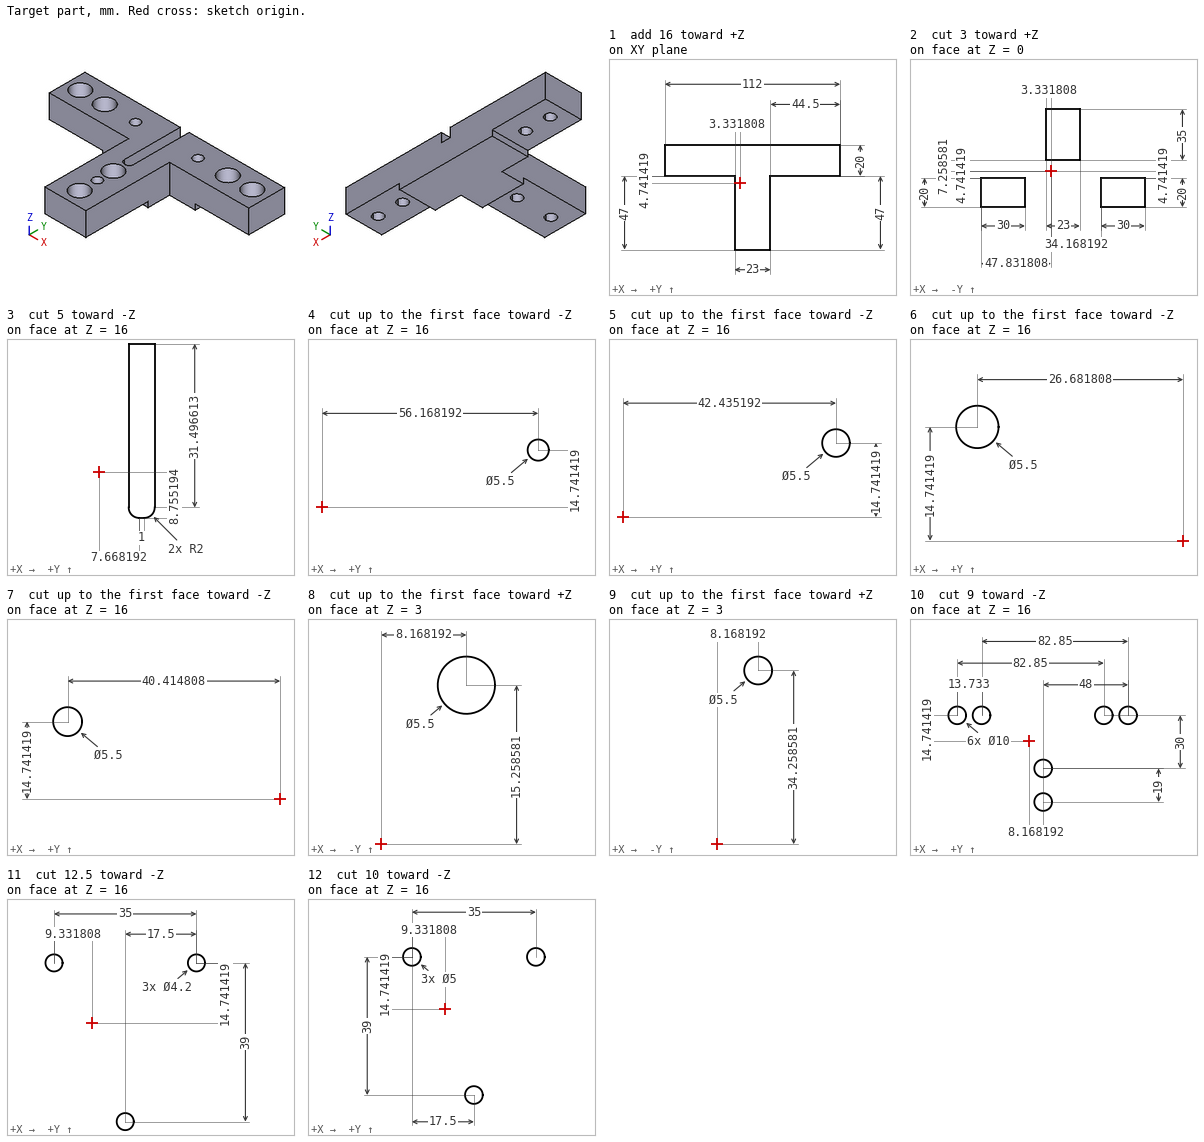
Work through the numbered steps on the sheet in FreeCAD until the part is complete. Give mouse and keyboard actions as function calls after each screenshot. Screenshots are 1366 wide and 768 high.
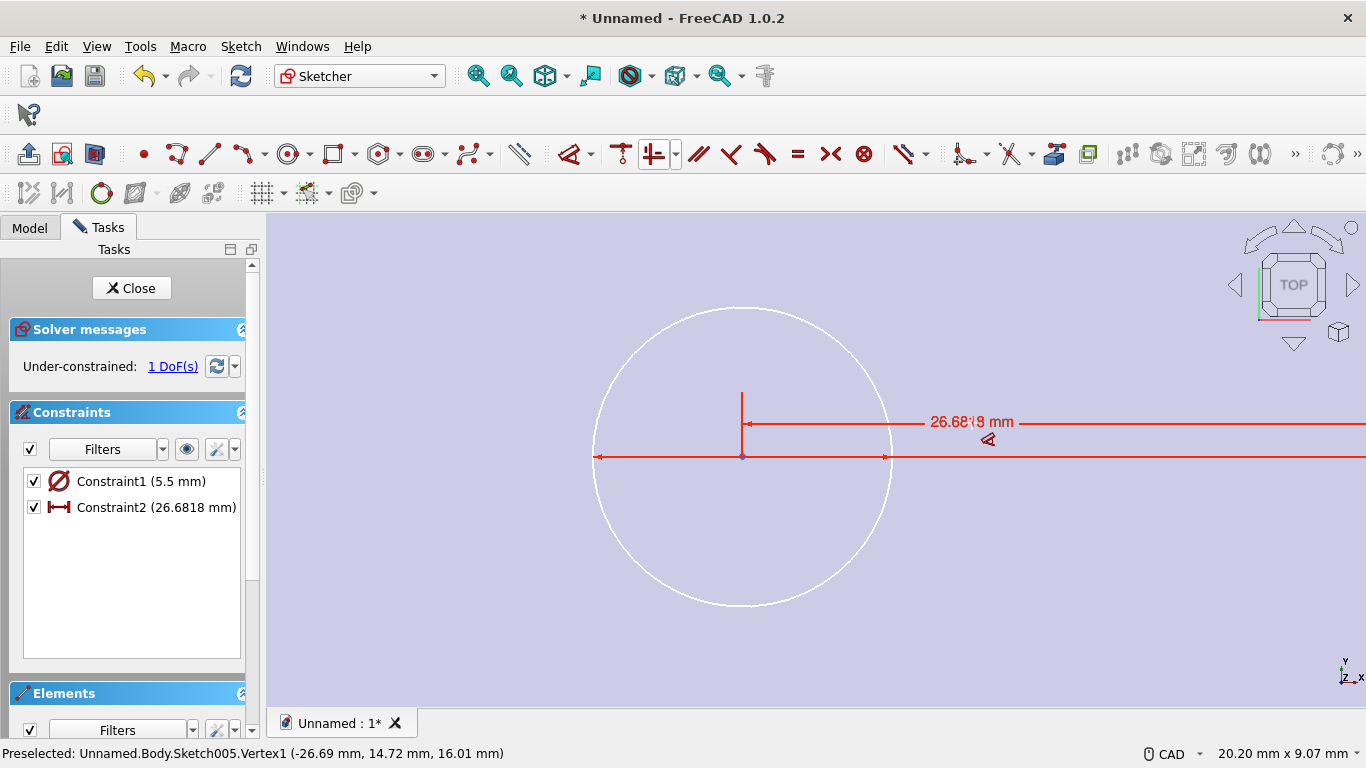
click(742, 457)
click(708, 568)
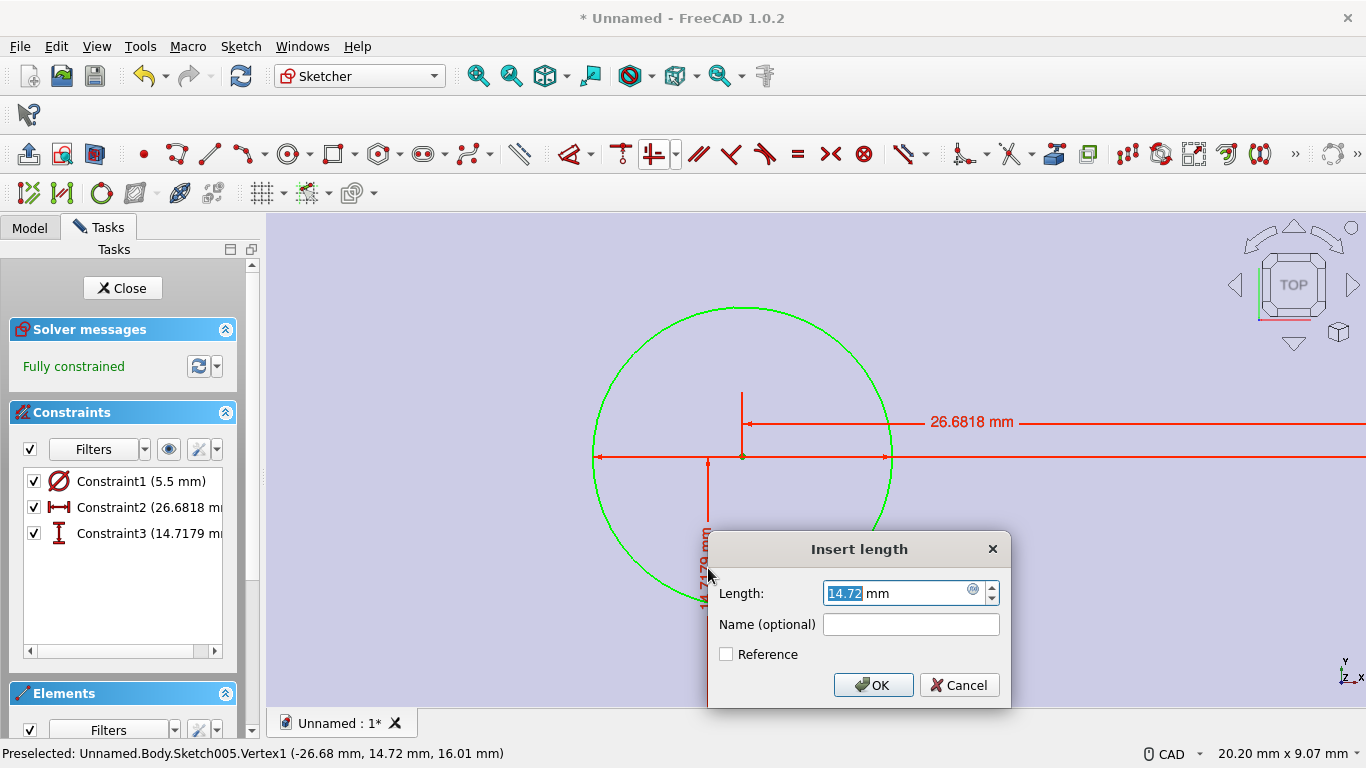
text(14.741419)
key(Return)
key(Escape)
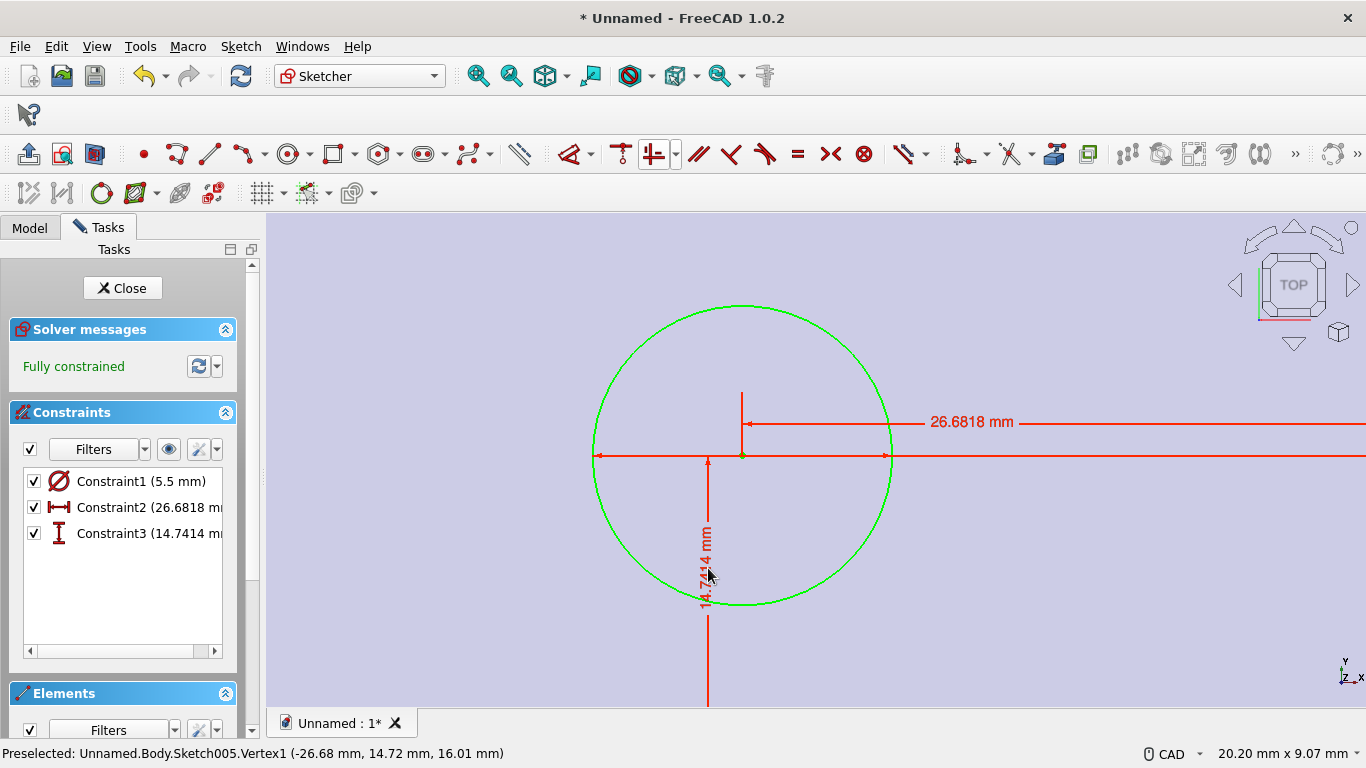
click(123, 288)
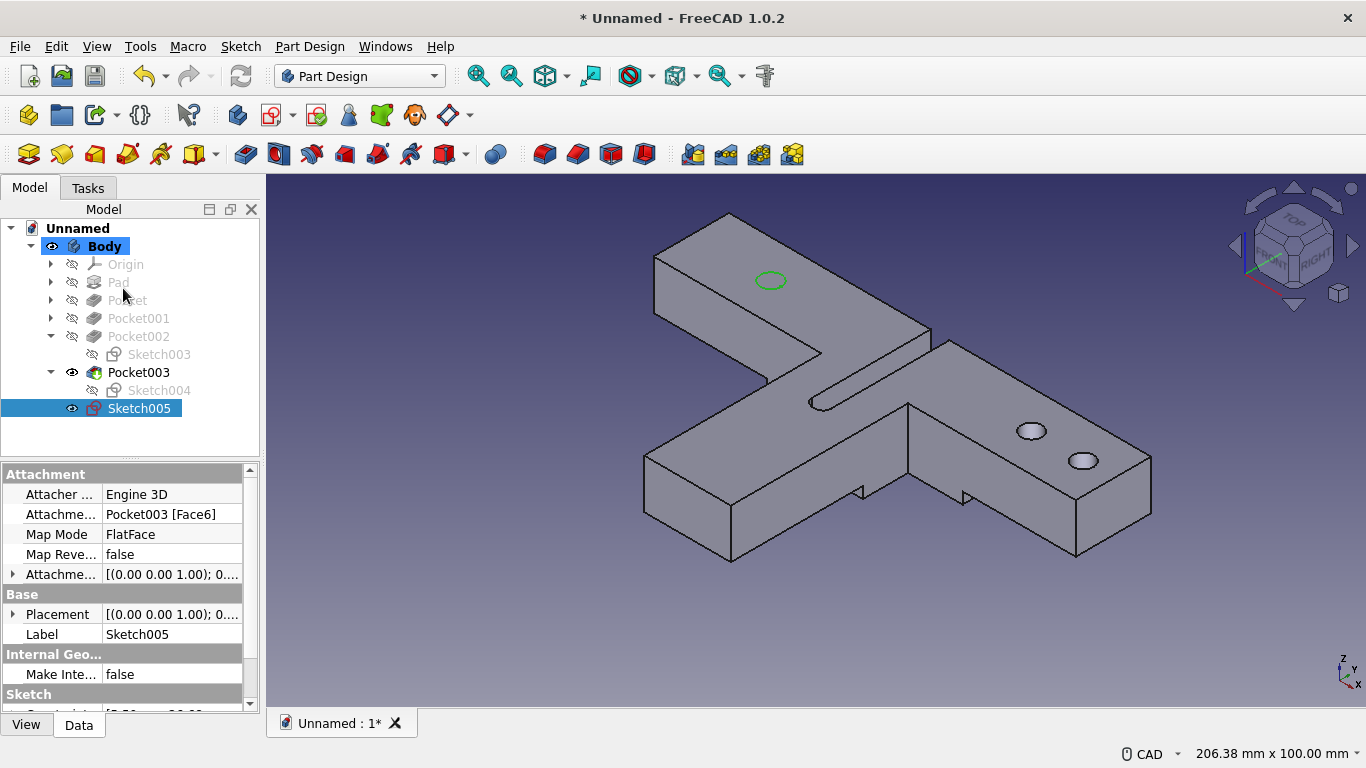
click(246, 154)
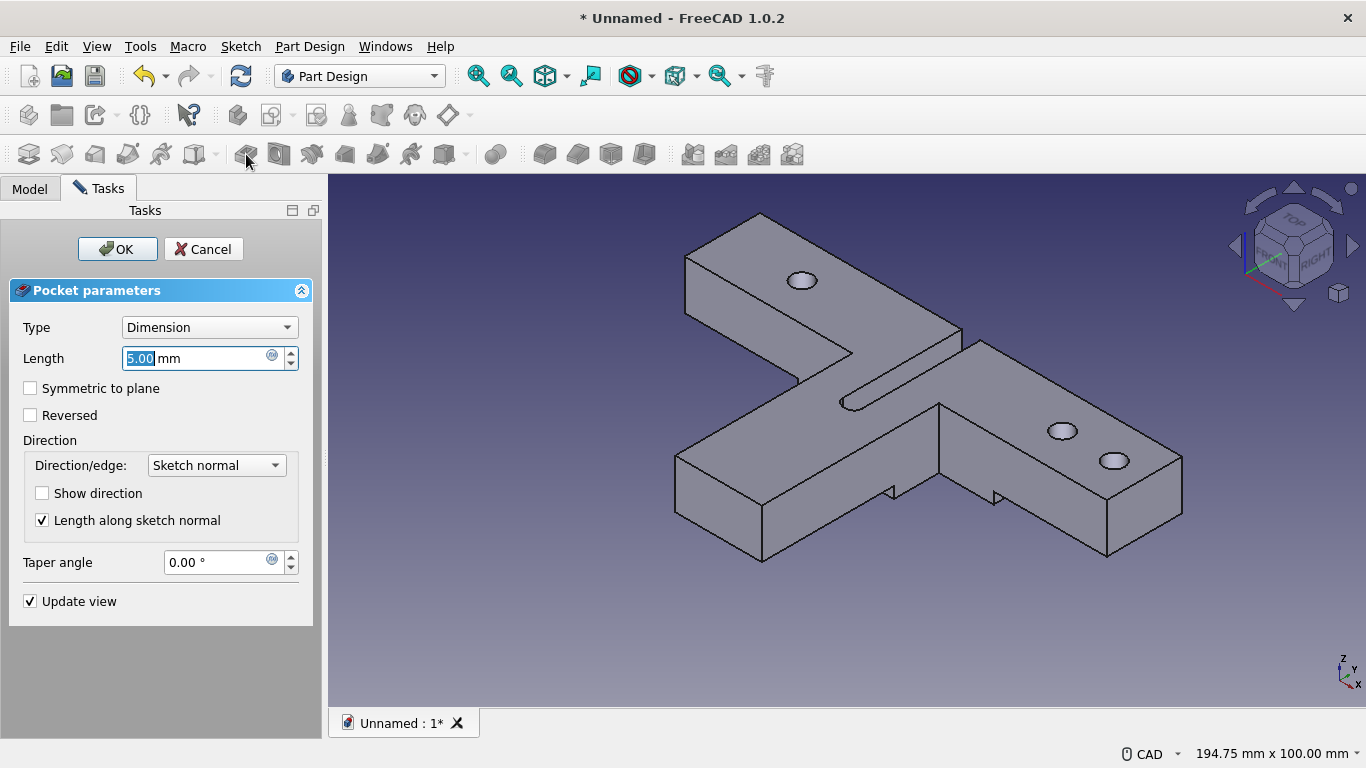
click(210, 328)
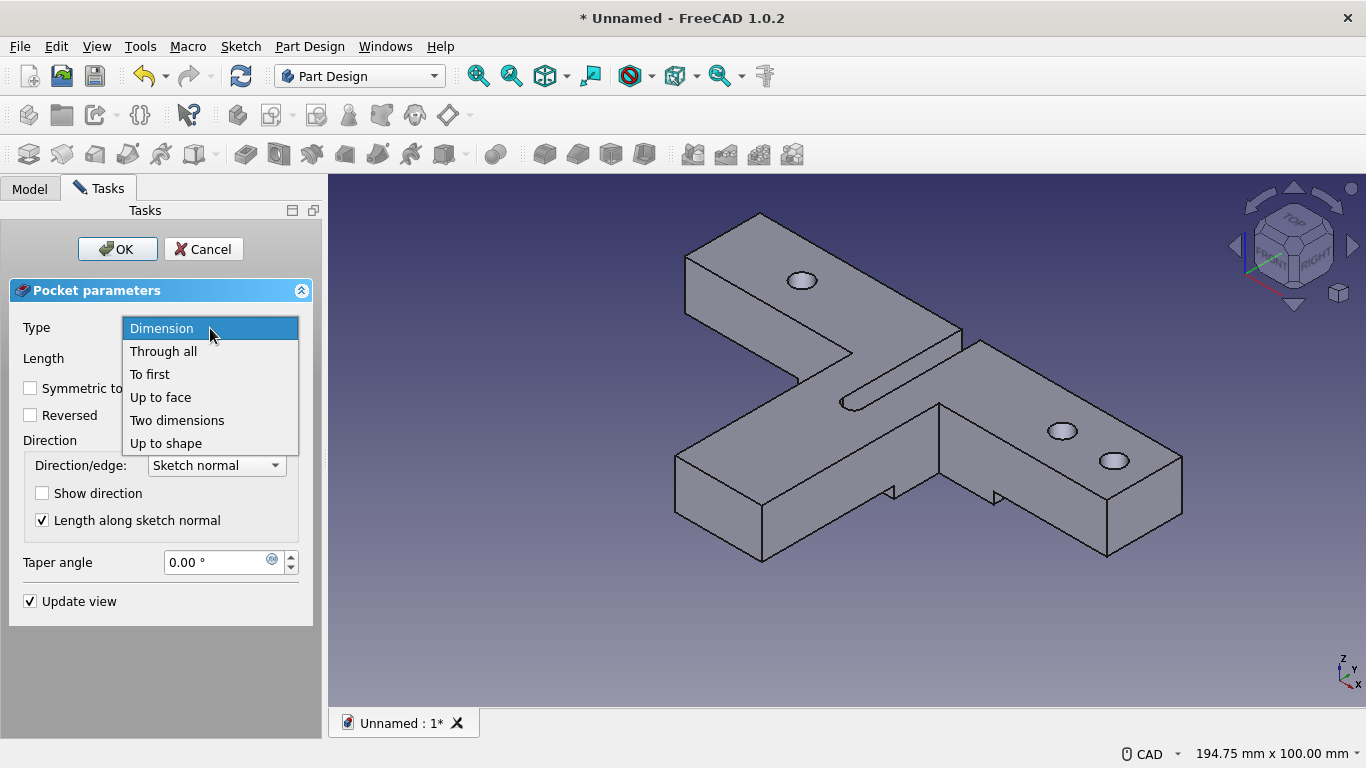
click(208, 374)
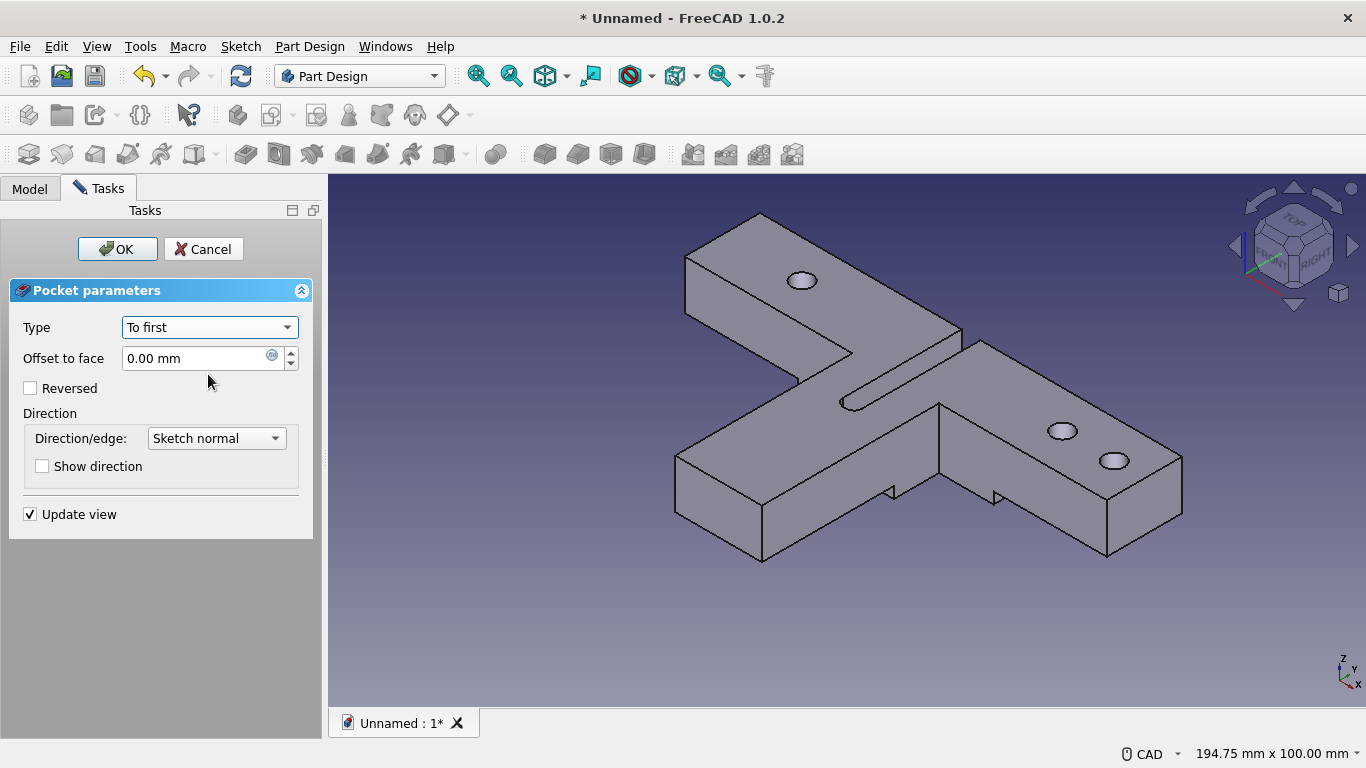
click(118, 249)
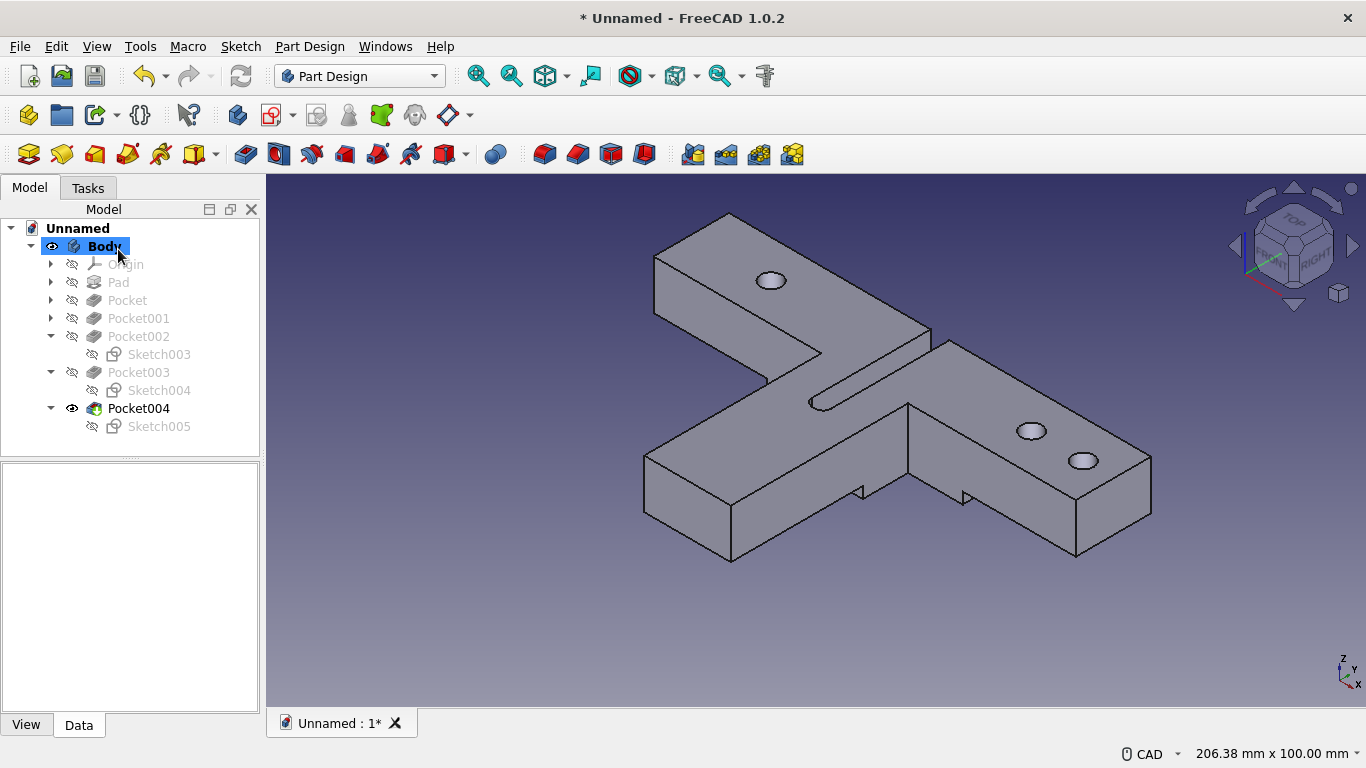
click(742, 448)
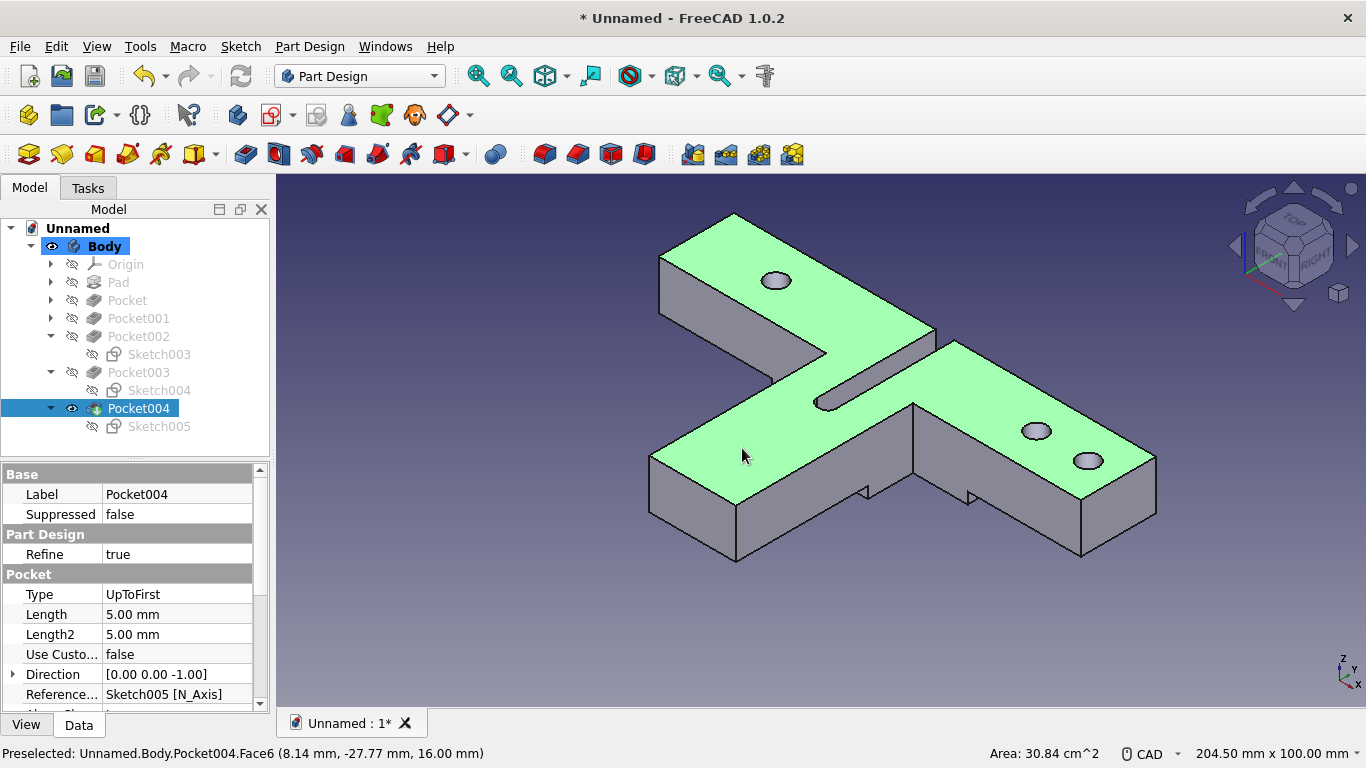
click(270, 116)